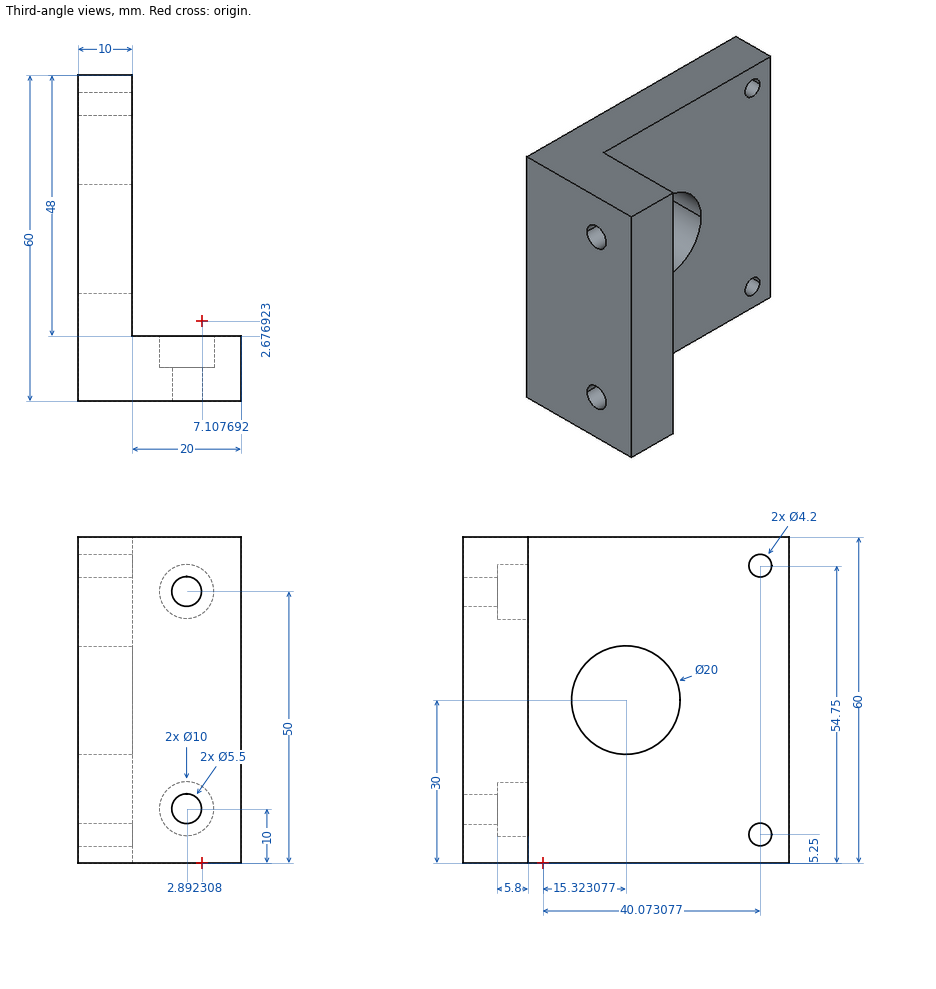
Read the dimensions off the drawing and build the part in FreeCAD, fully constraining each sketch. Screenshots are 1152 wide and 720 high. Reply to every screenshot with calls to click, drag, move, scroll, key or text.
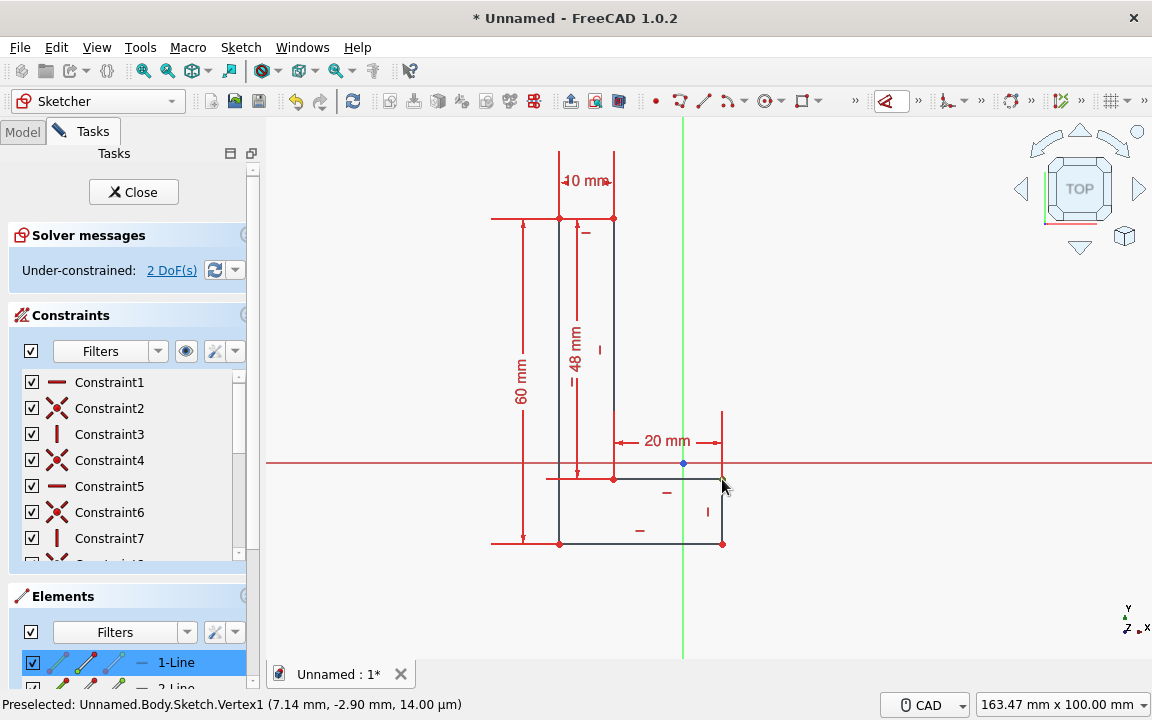
key(l)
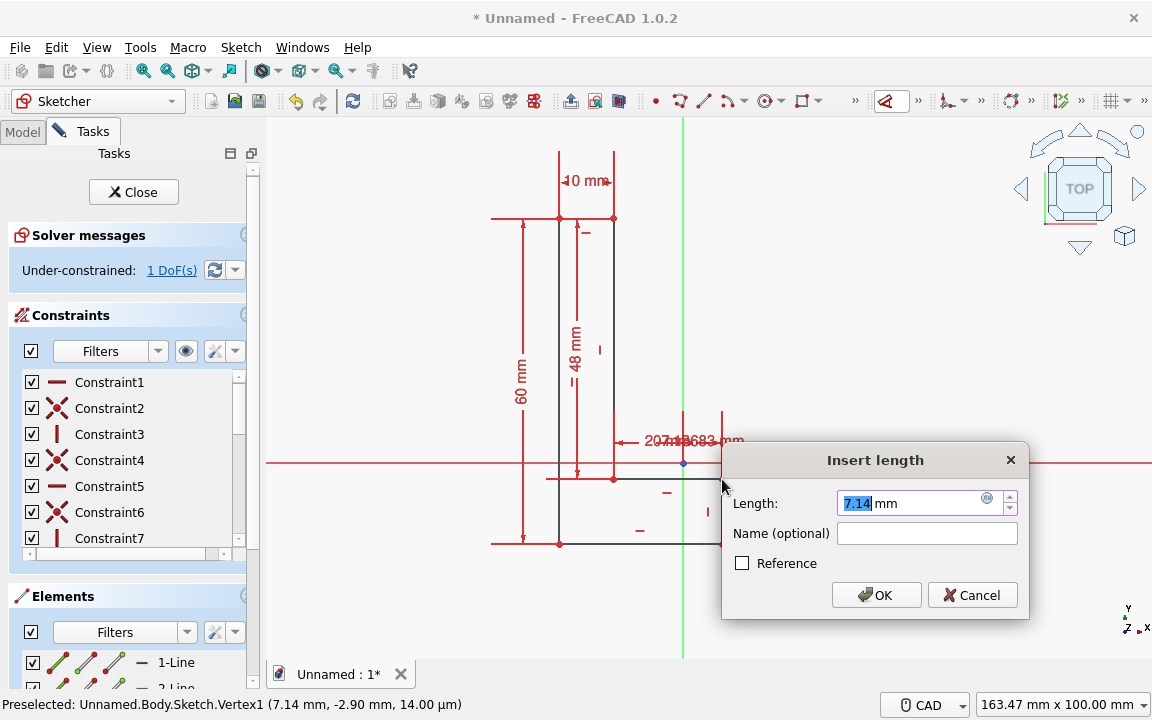
text(7.107692)
key(Return)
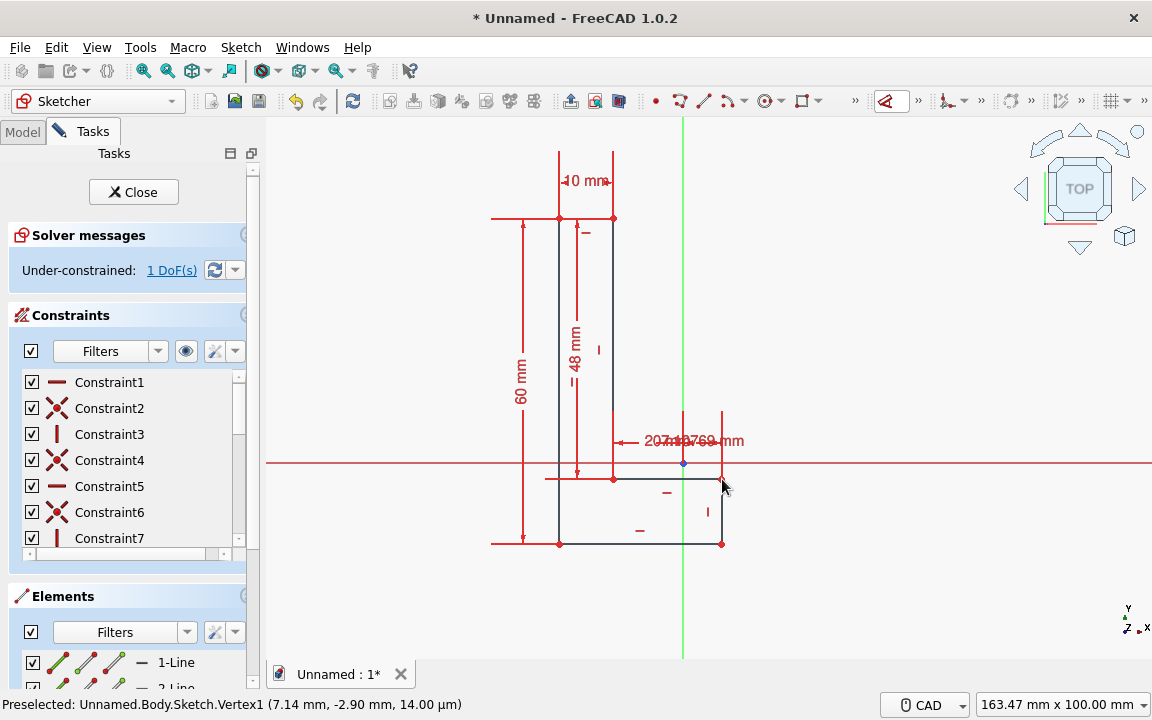
scroll(722, 479, up, 6)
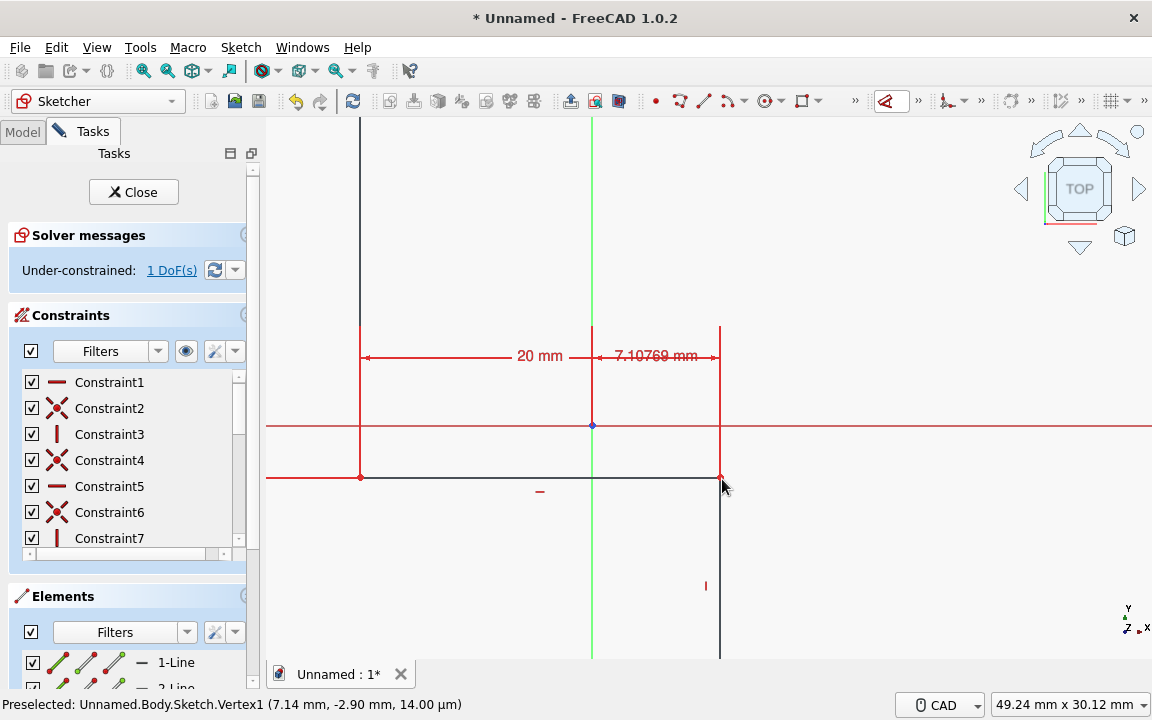
click(720, 478)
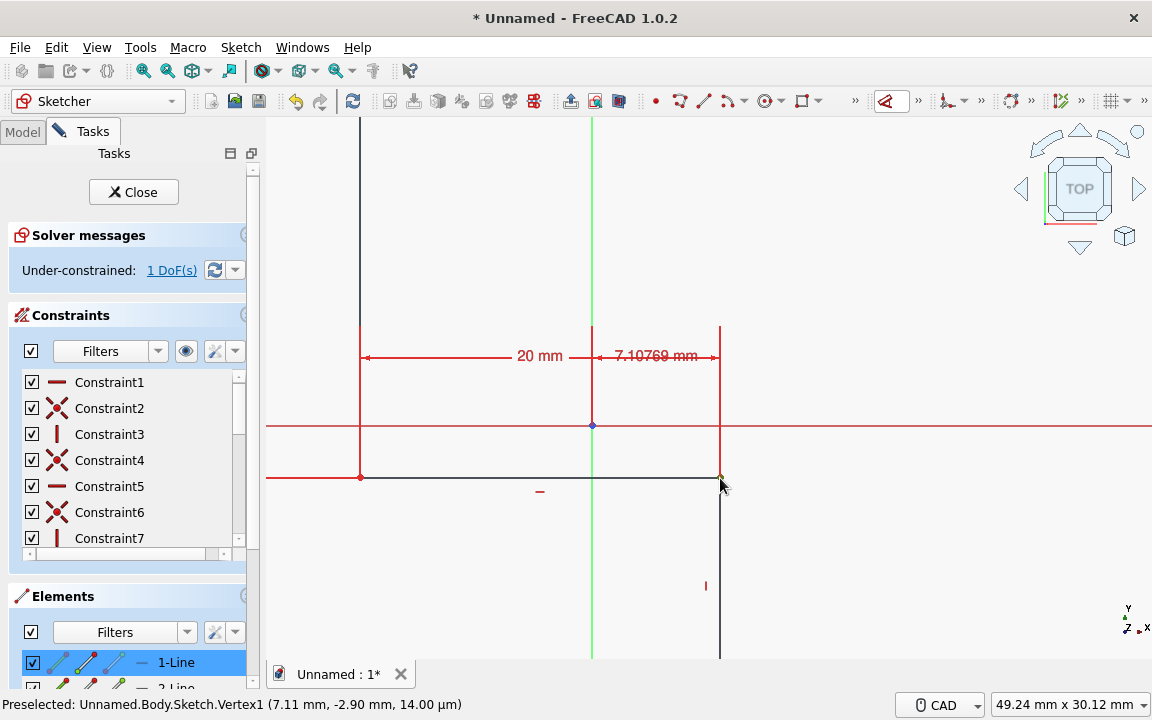
click(904, 102)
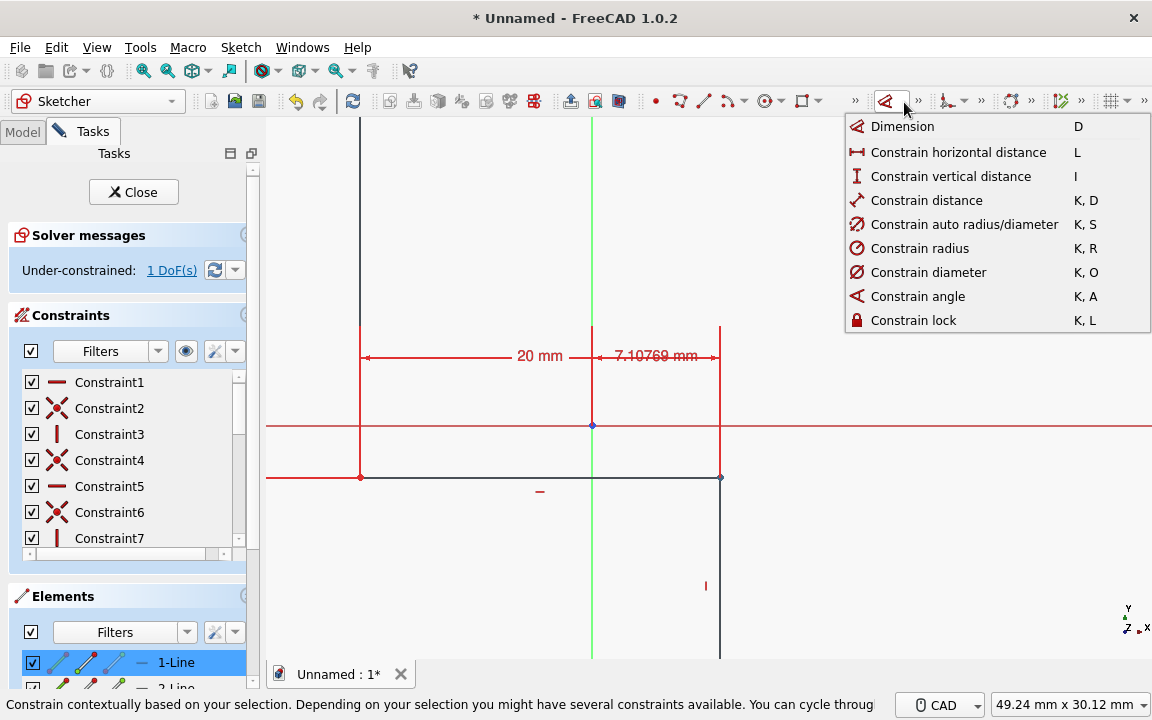
click(998, 176)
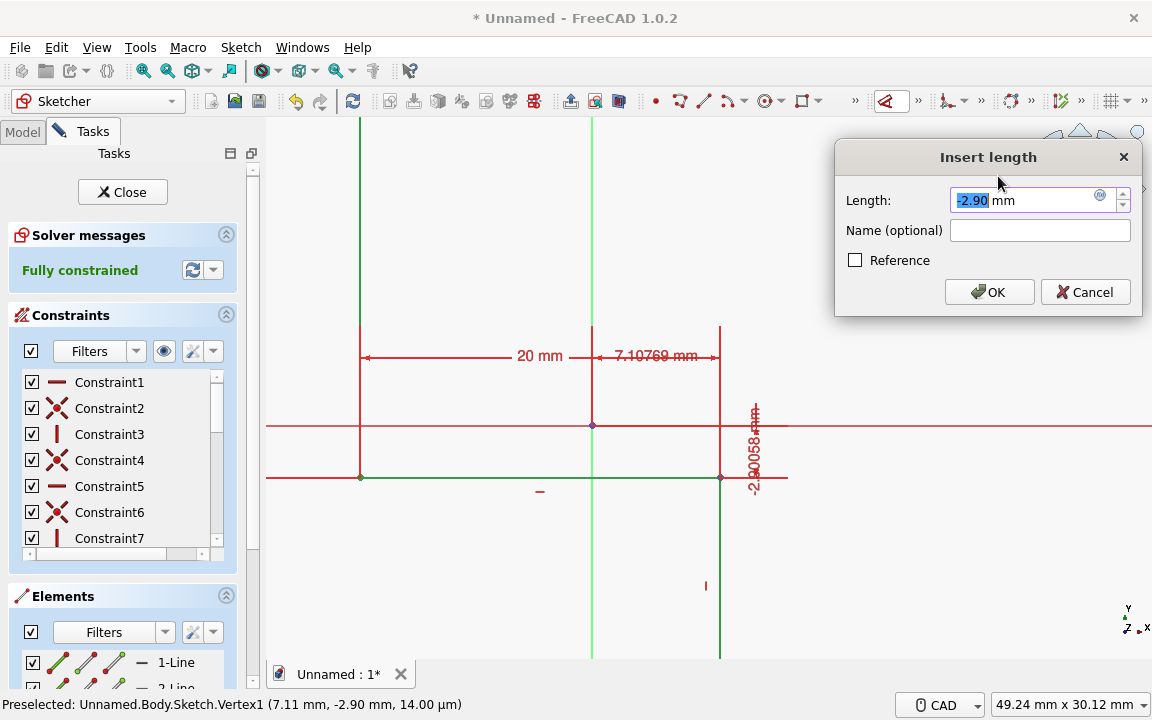
text(-2.676923)
key(Return)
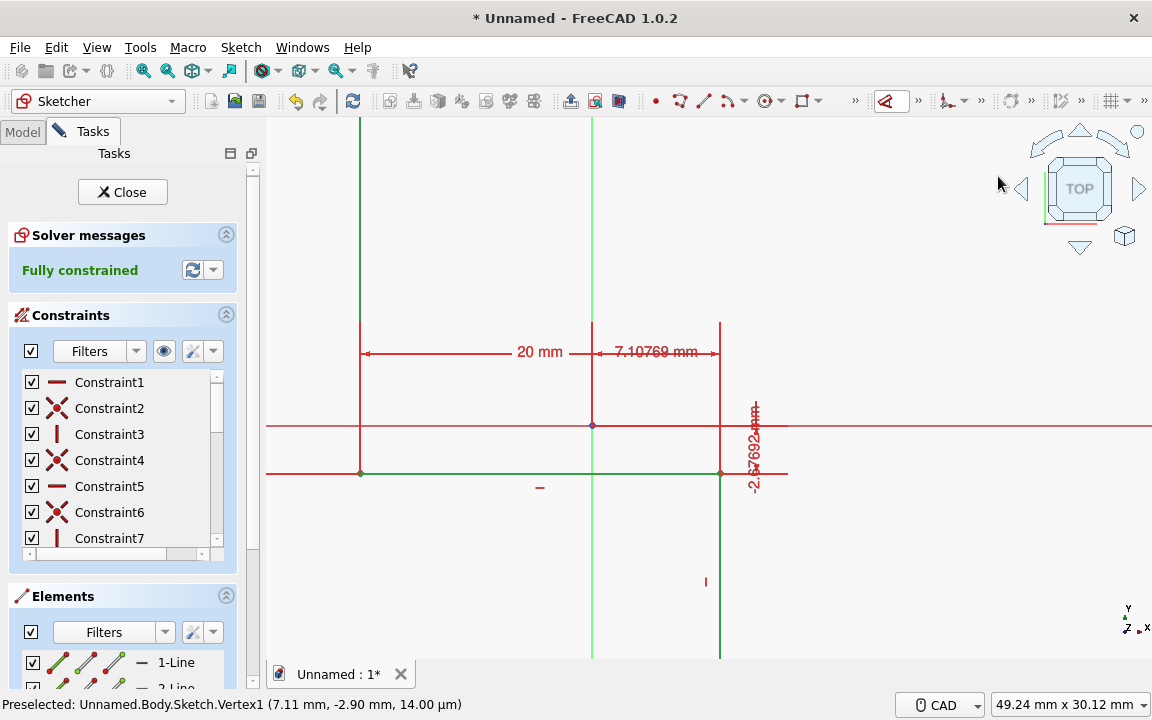
click(123, 192)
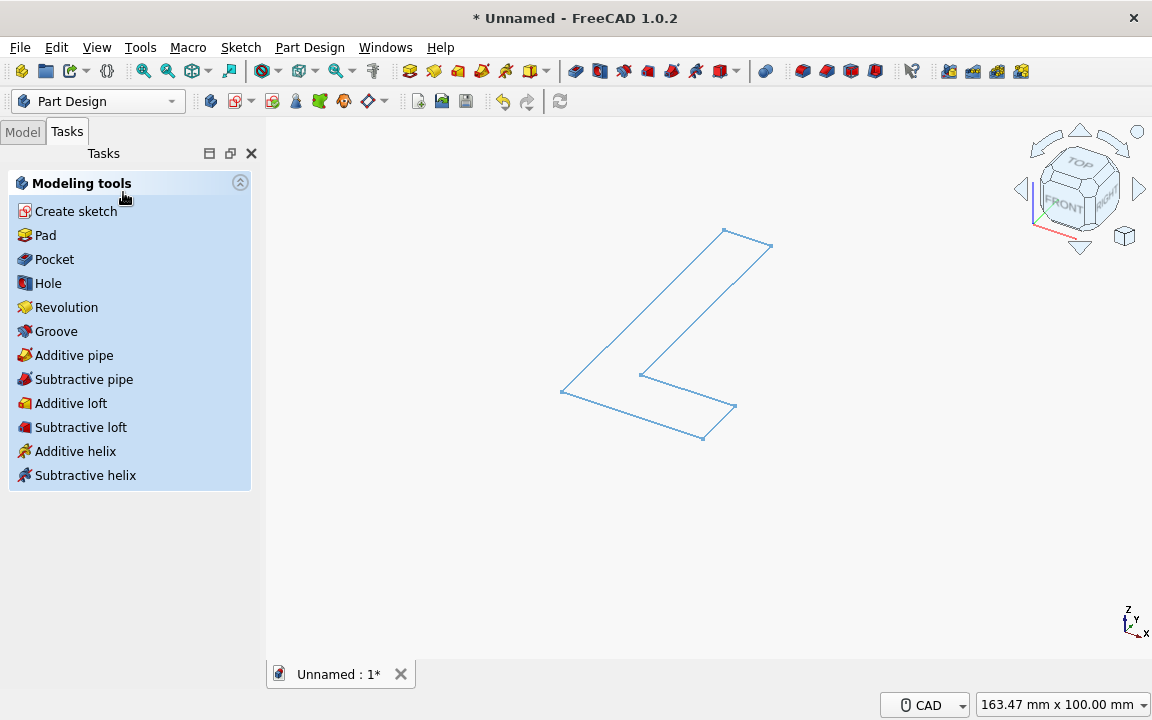
click(410, 72)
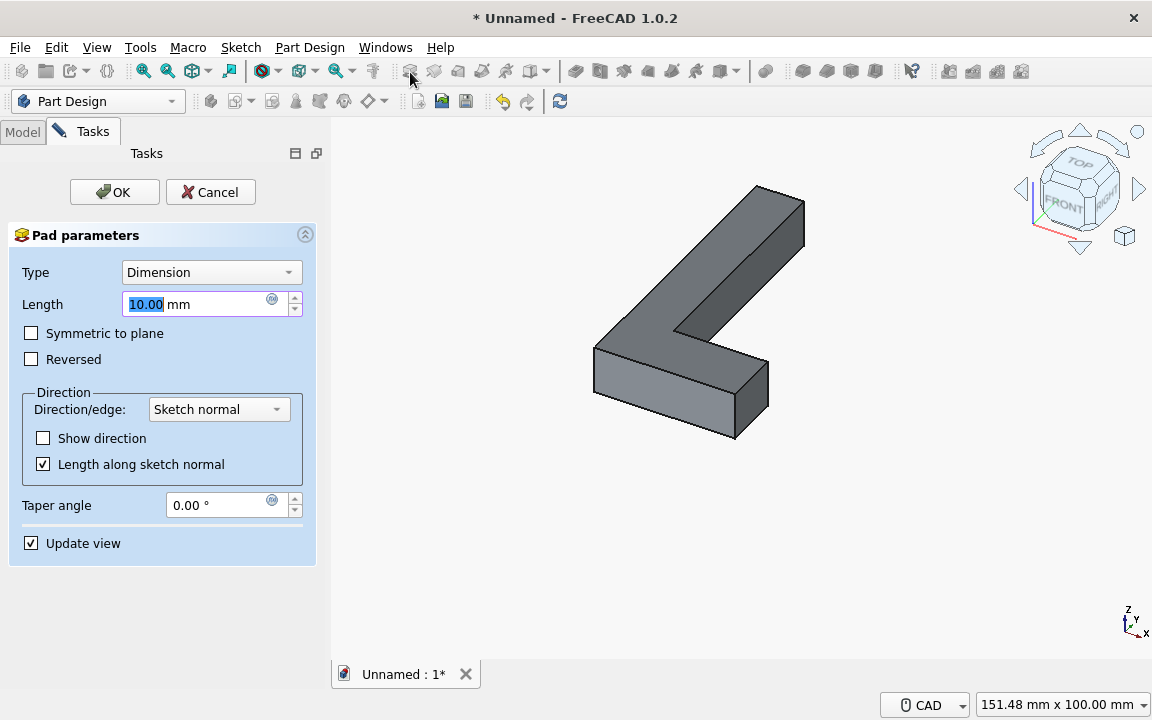
text(60)
key(Tab)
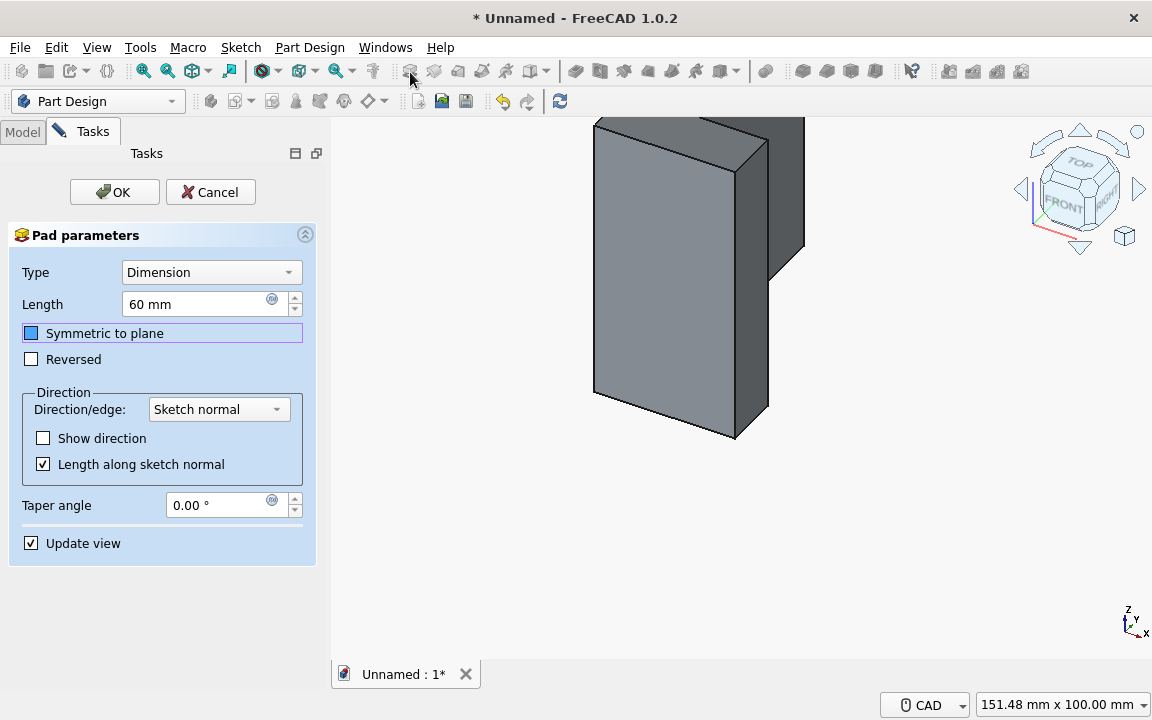
click(115, 192)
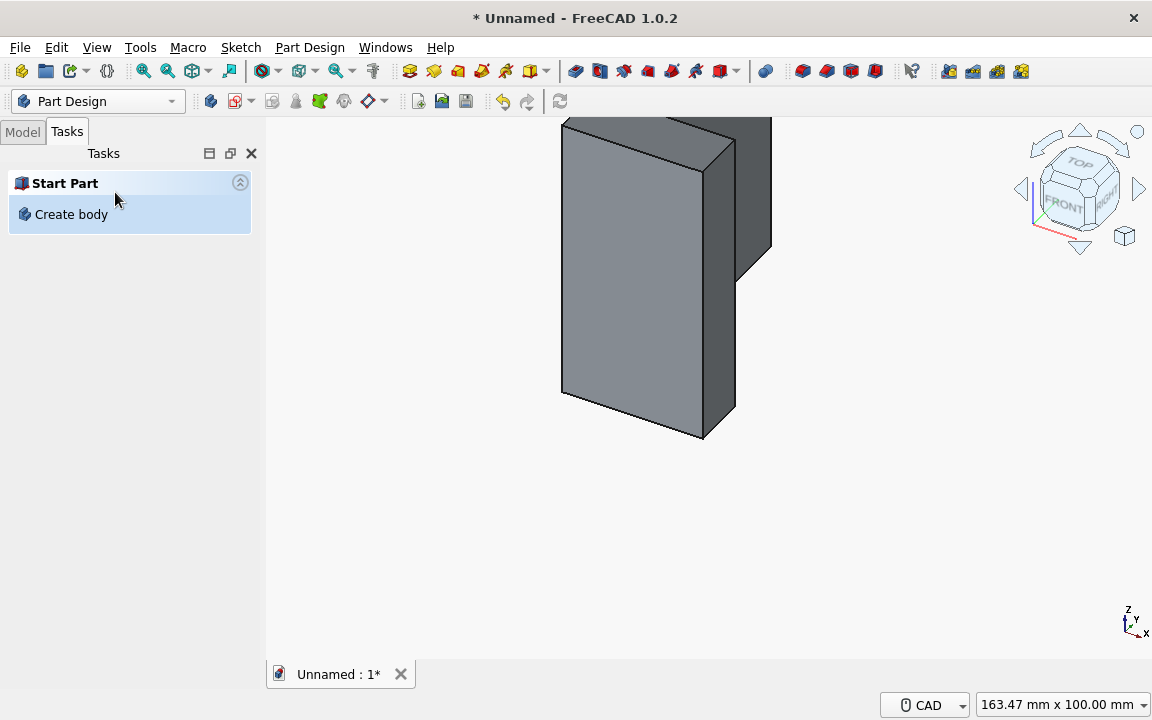
click(144, 72)